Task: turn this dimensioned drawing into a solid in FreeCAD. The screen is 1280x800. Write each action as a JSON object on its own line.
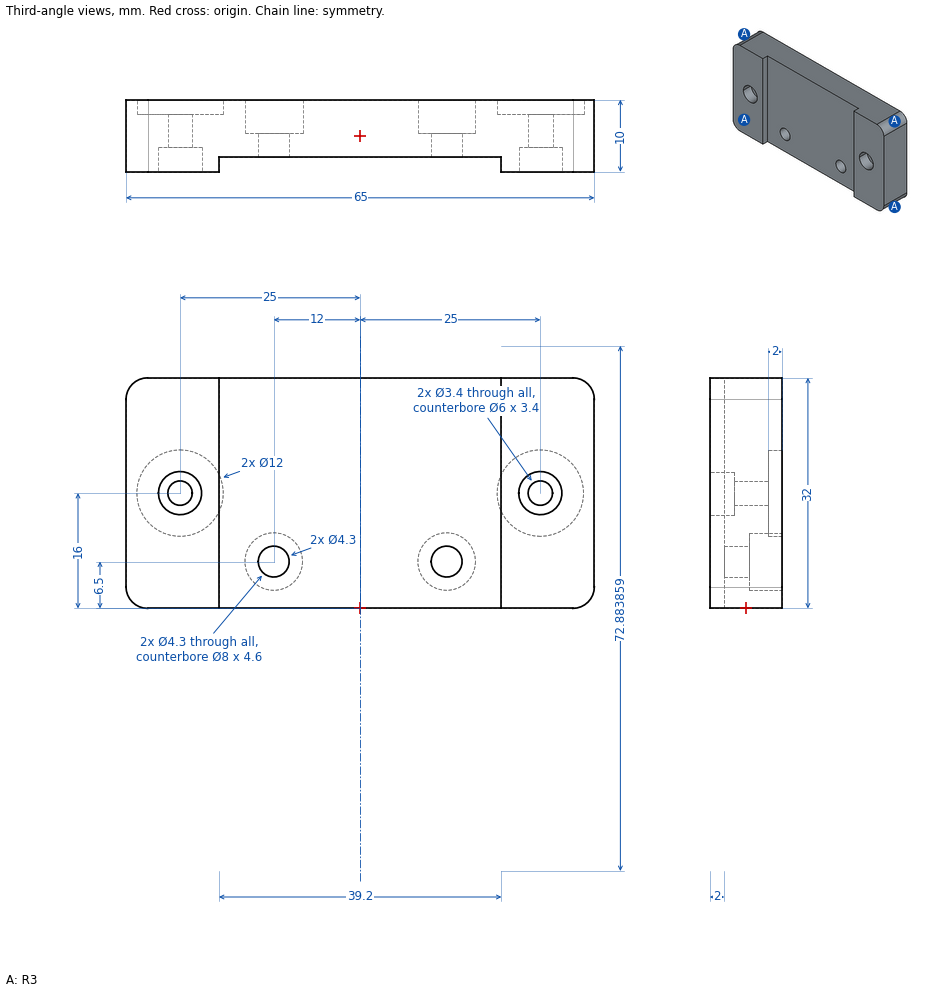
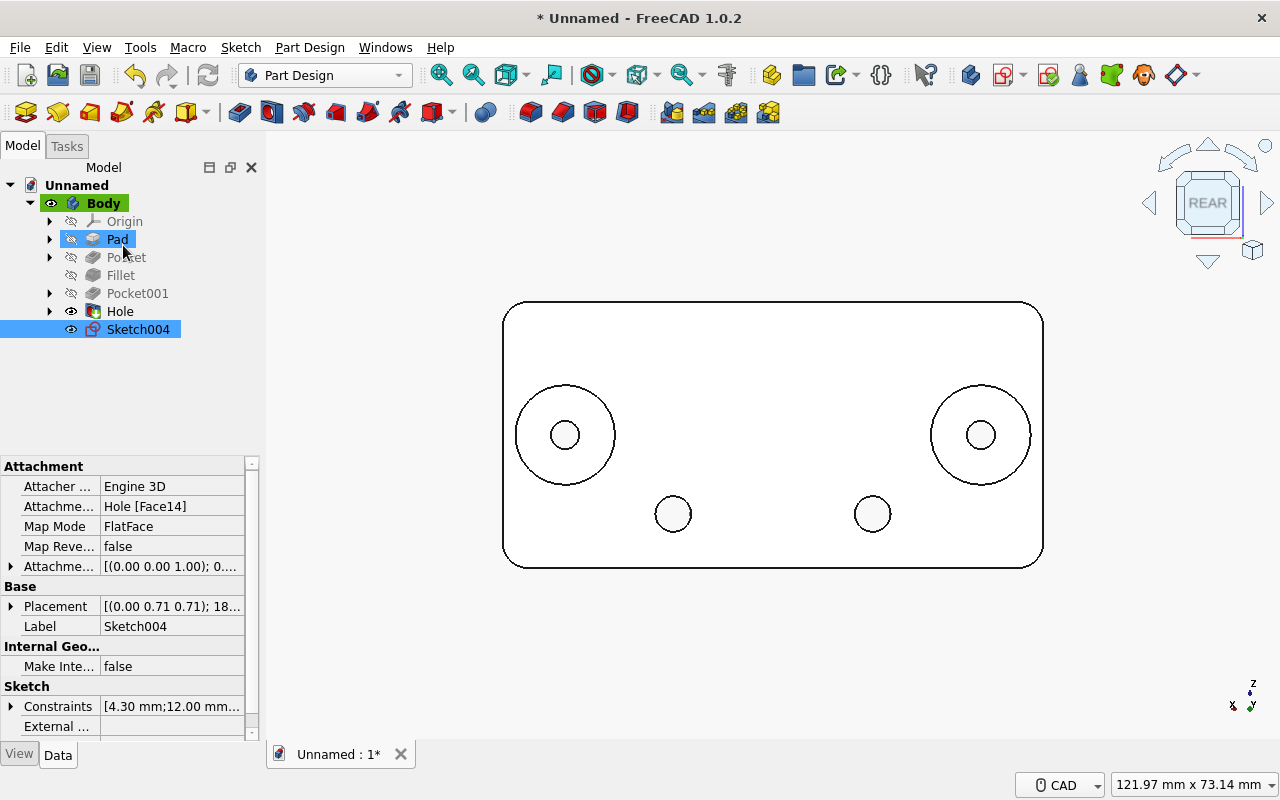
{"action": "left_click", "coordinate": [272, 112]}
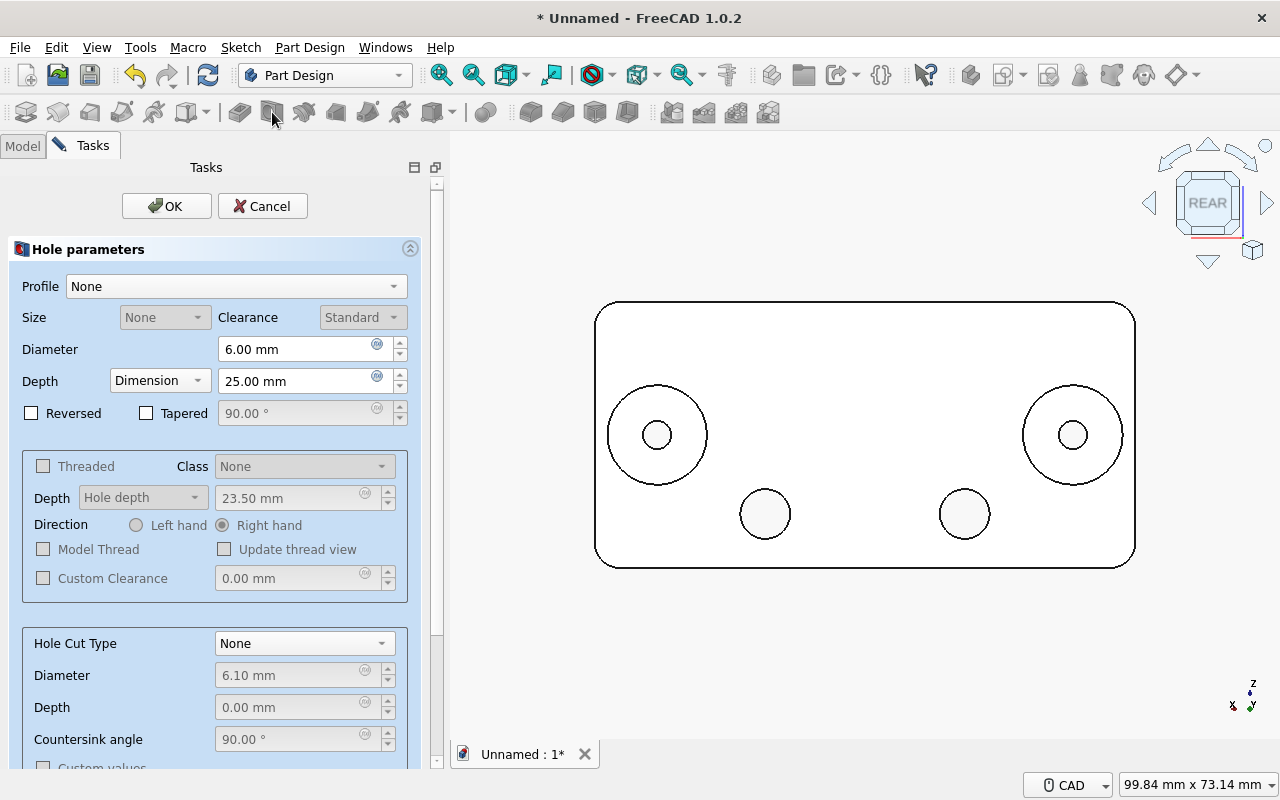
{"action": "triple_click", "coordinate": [305, 349]}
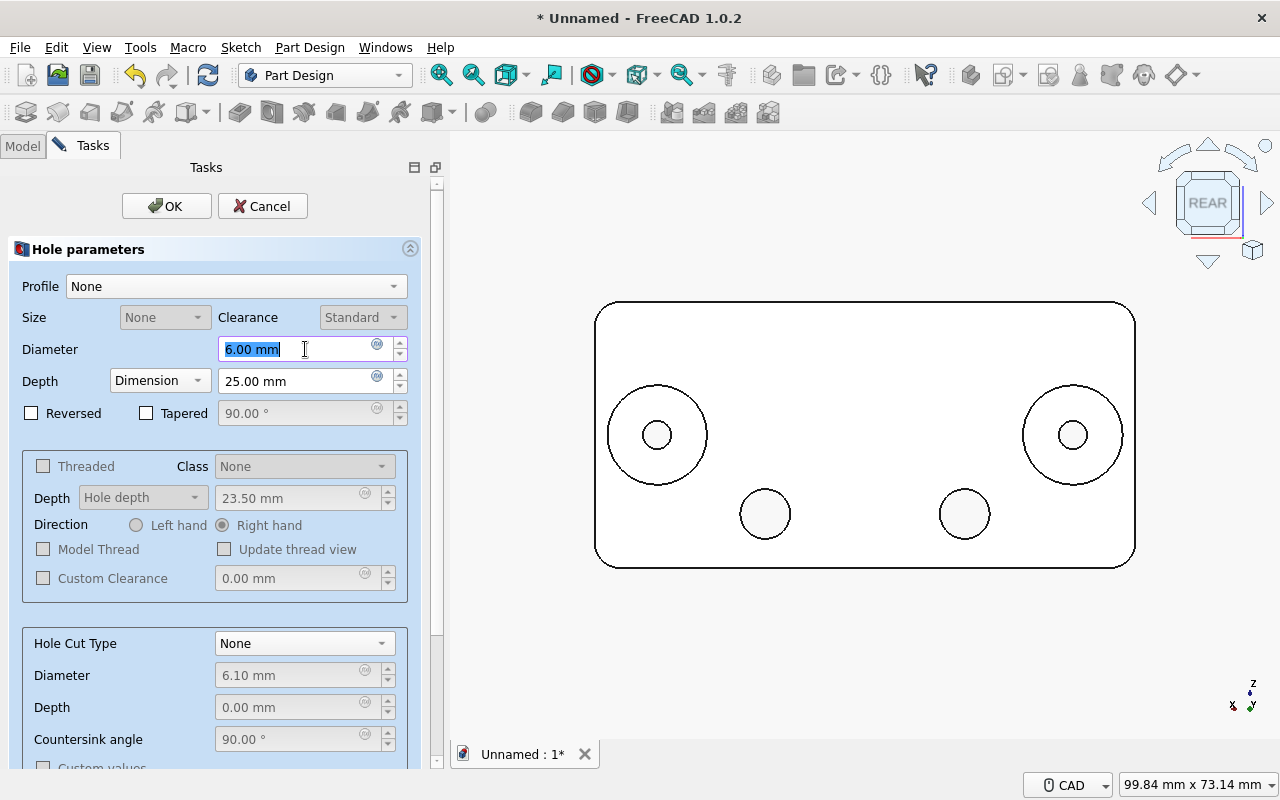
{"action": "type", "text": "4.3"}
{"action": "key", "text": "Tab"}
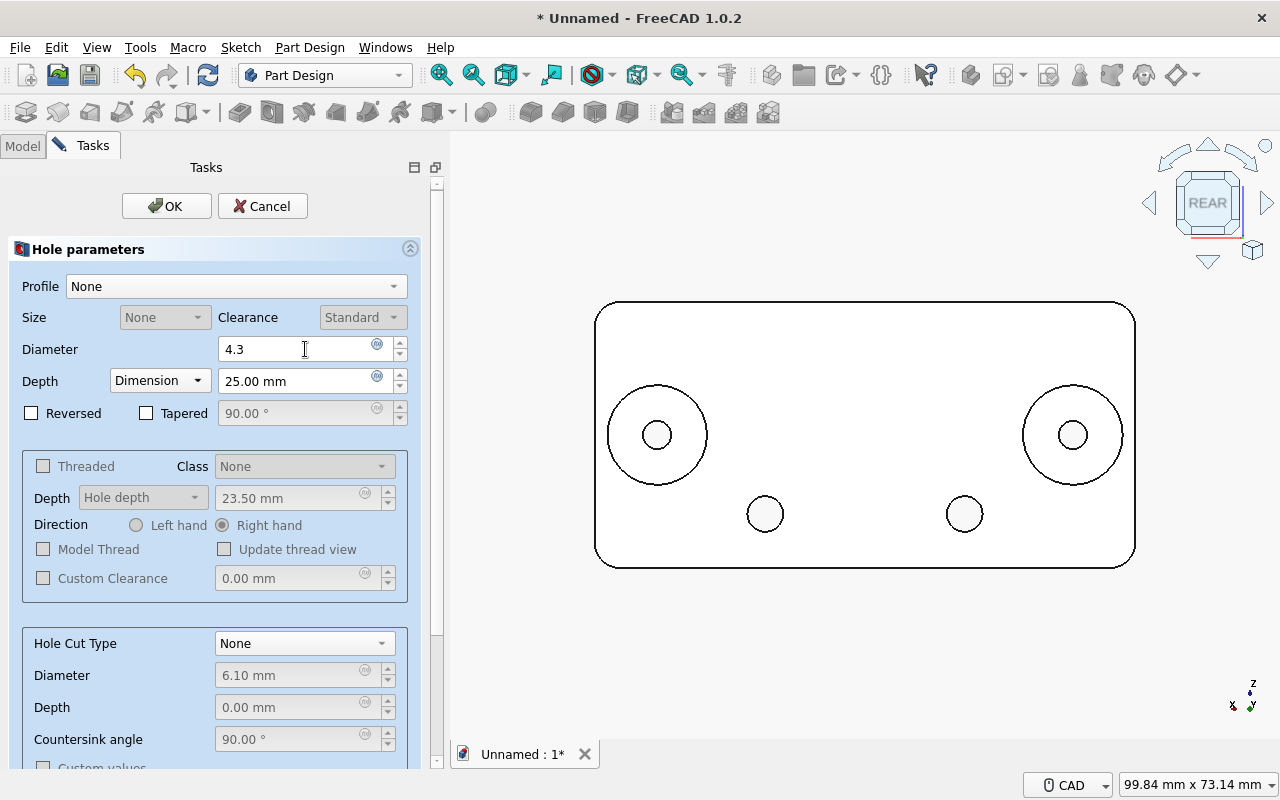
{"action": "left_click", "coordinate": [161, 380]}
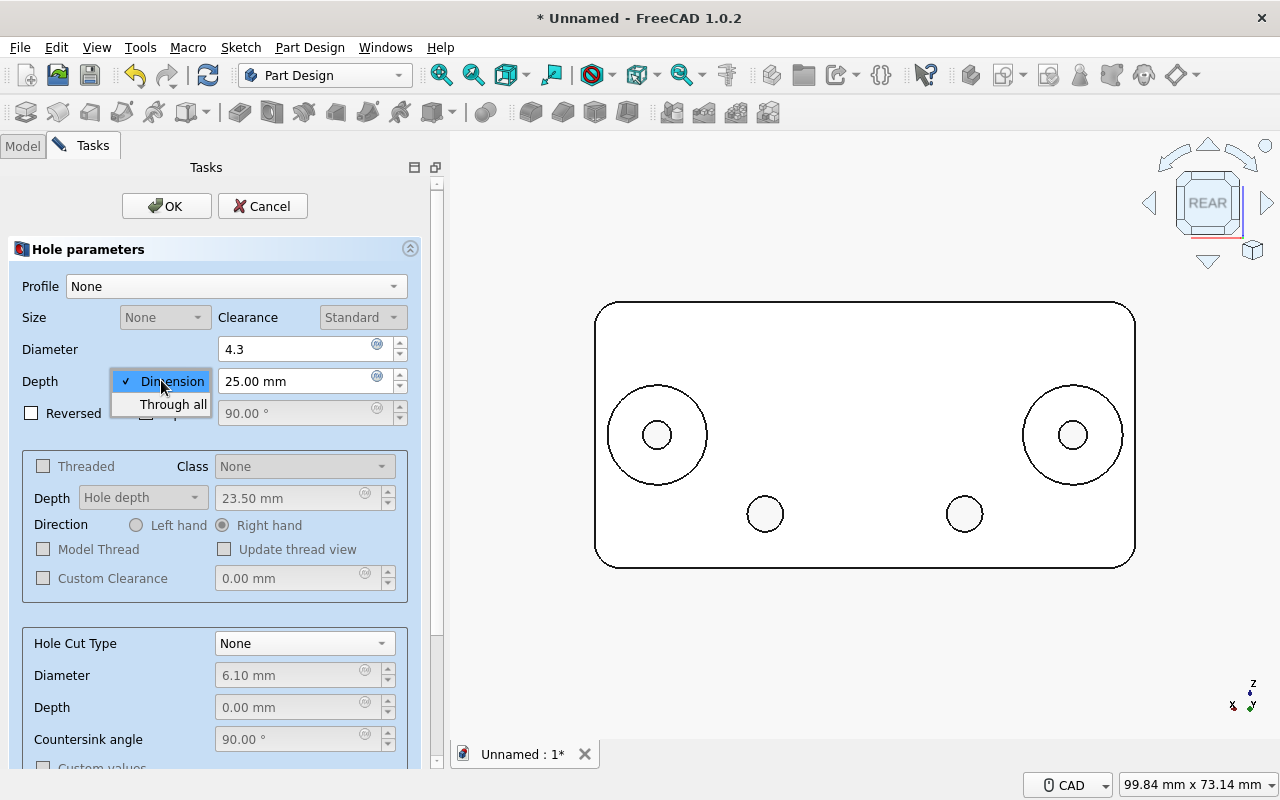
{"action": "left_click", "coordinate": [160, 404]}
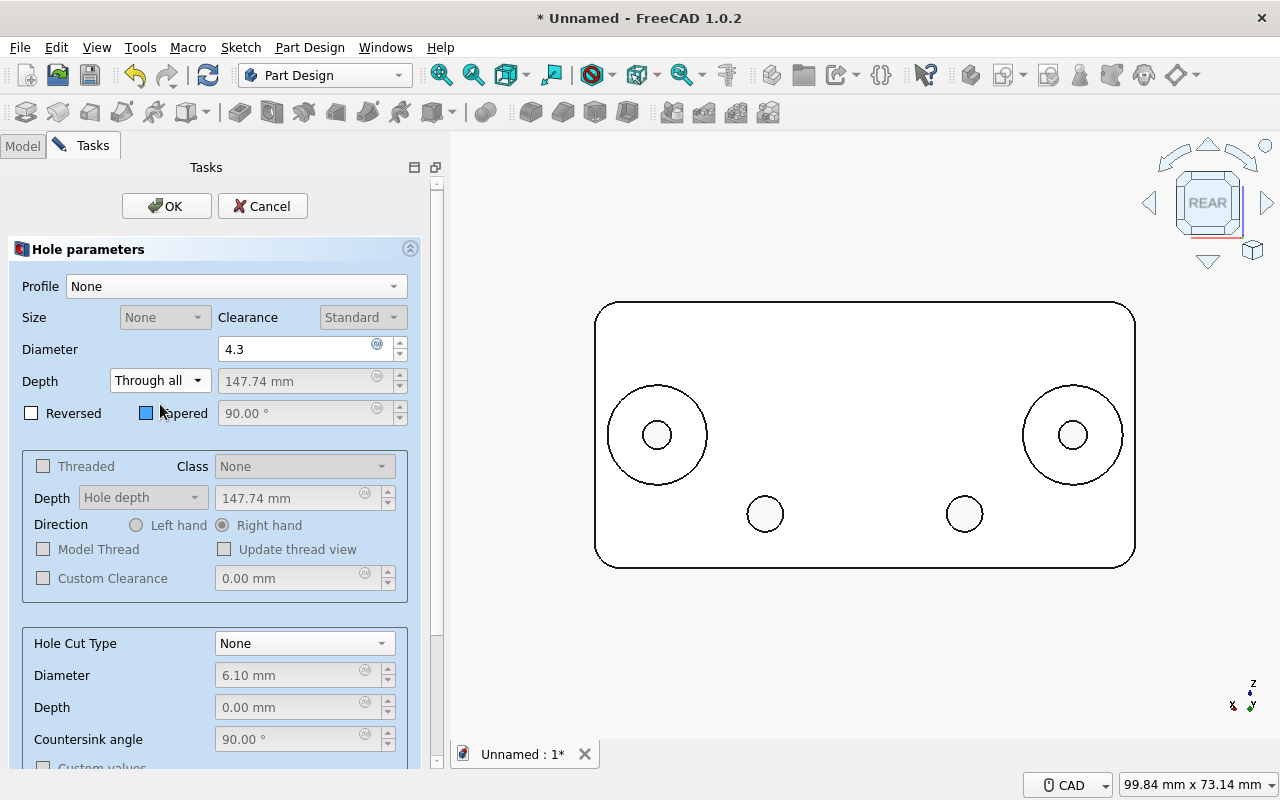
{"action": "left_click", "coordinate": [306, 644]}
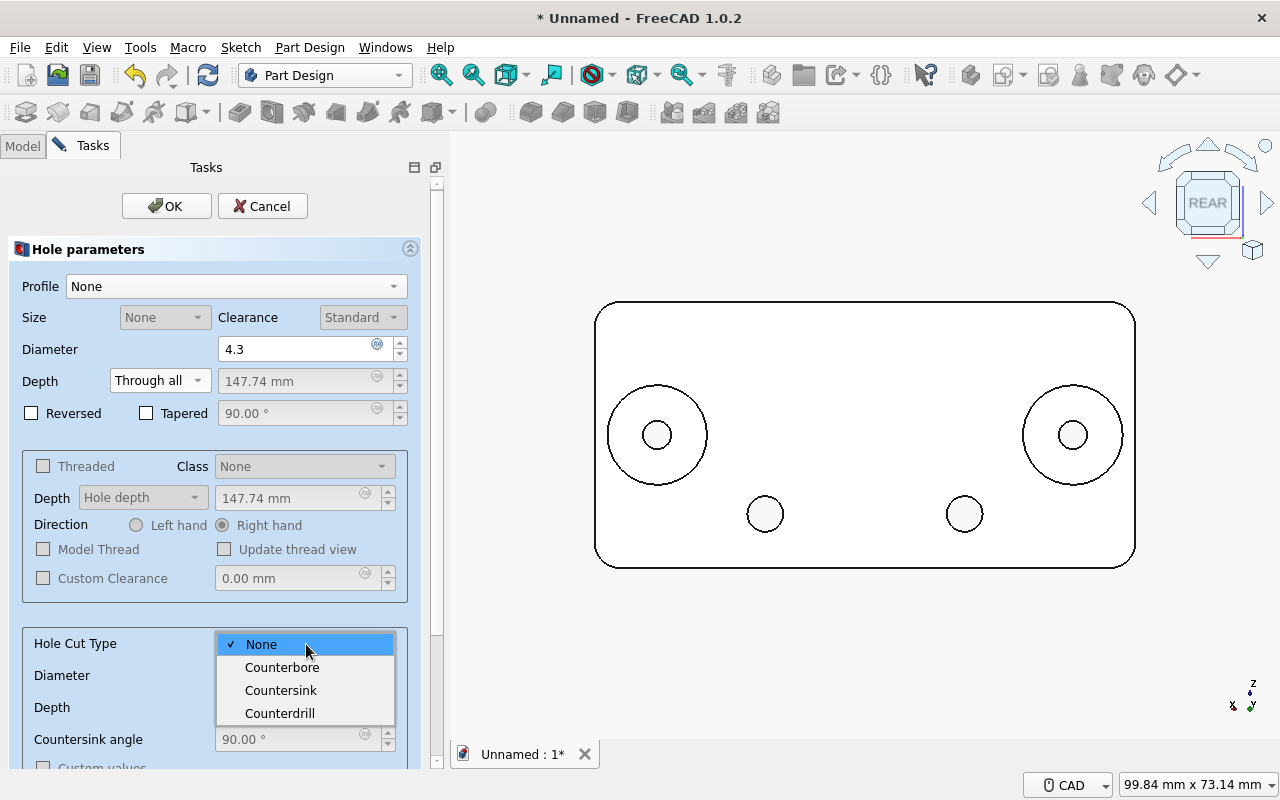
{"action": "left_click", "coordinate": [304, 668]}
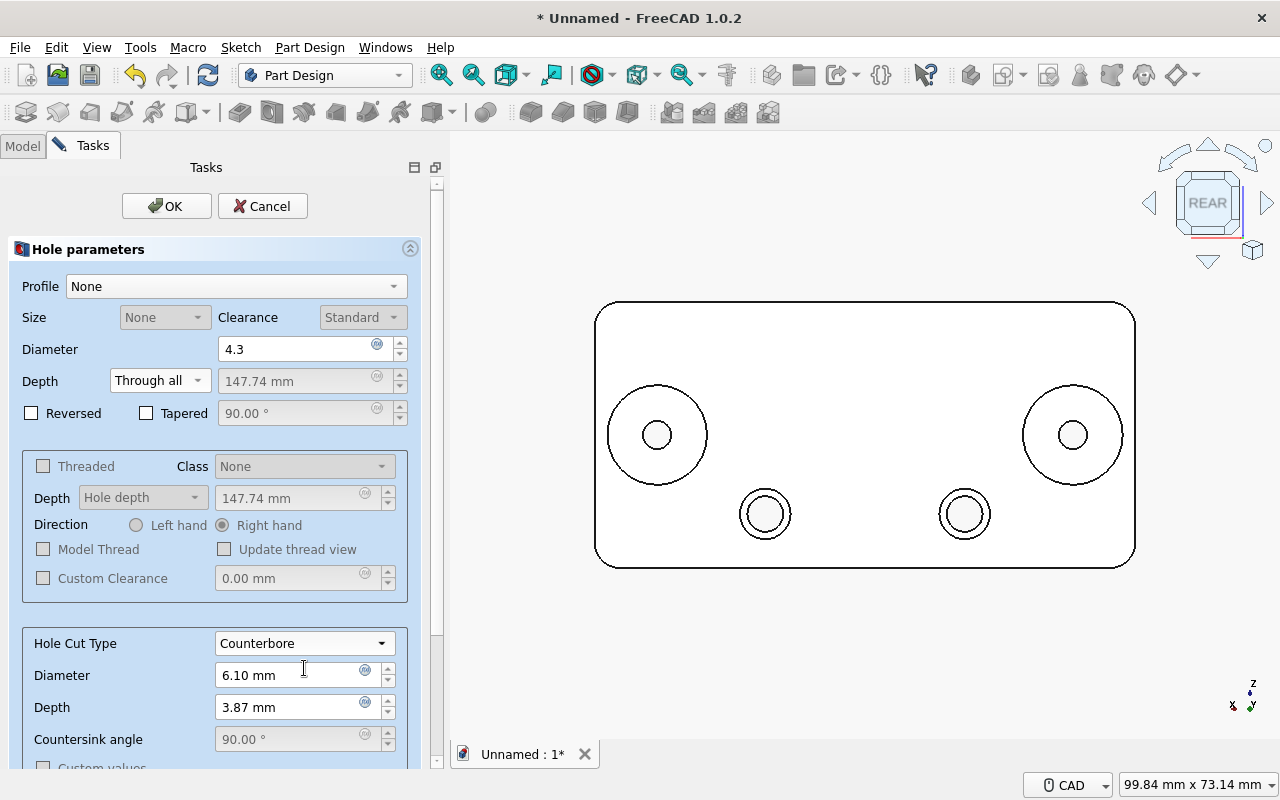
{"action": "triple_click", "coordinate": [298, 675]}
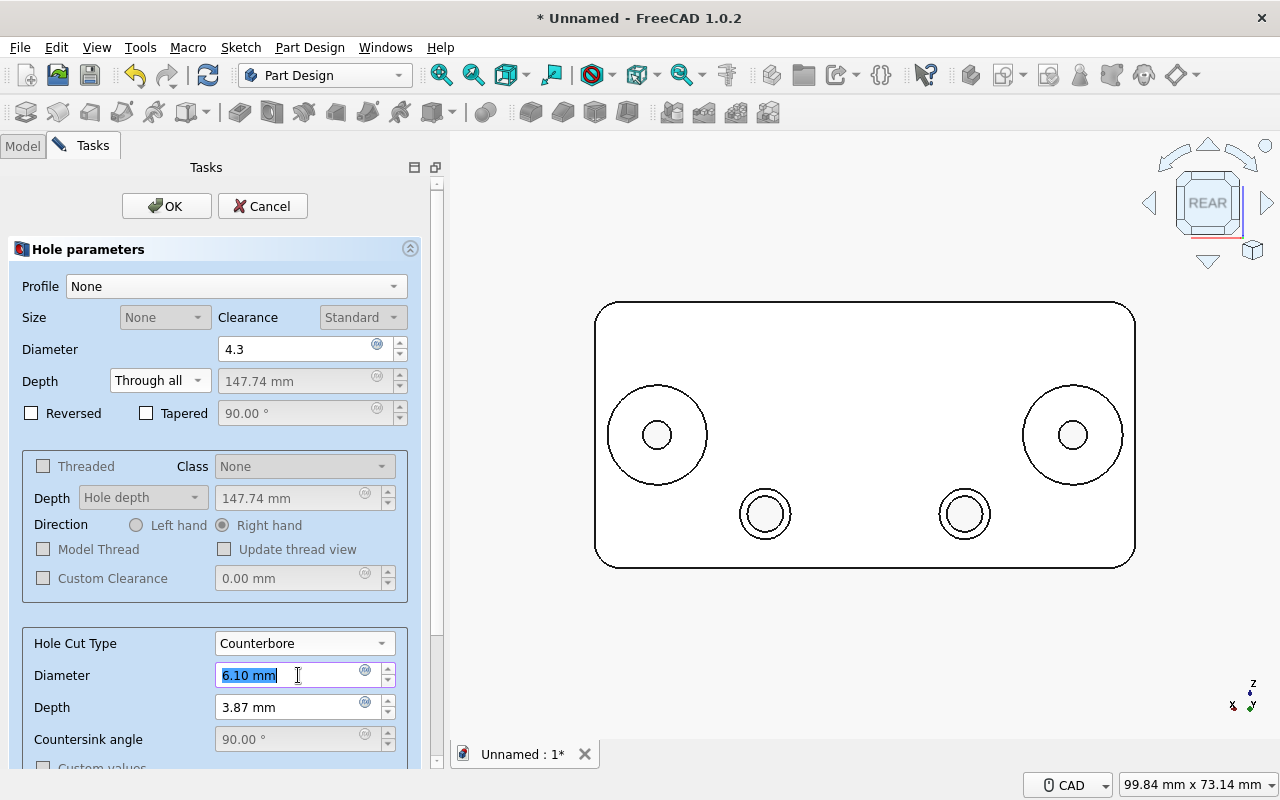
{"action": "type", "text": "8"}
{"action": "key", "text": "Tab"}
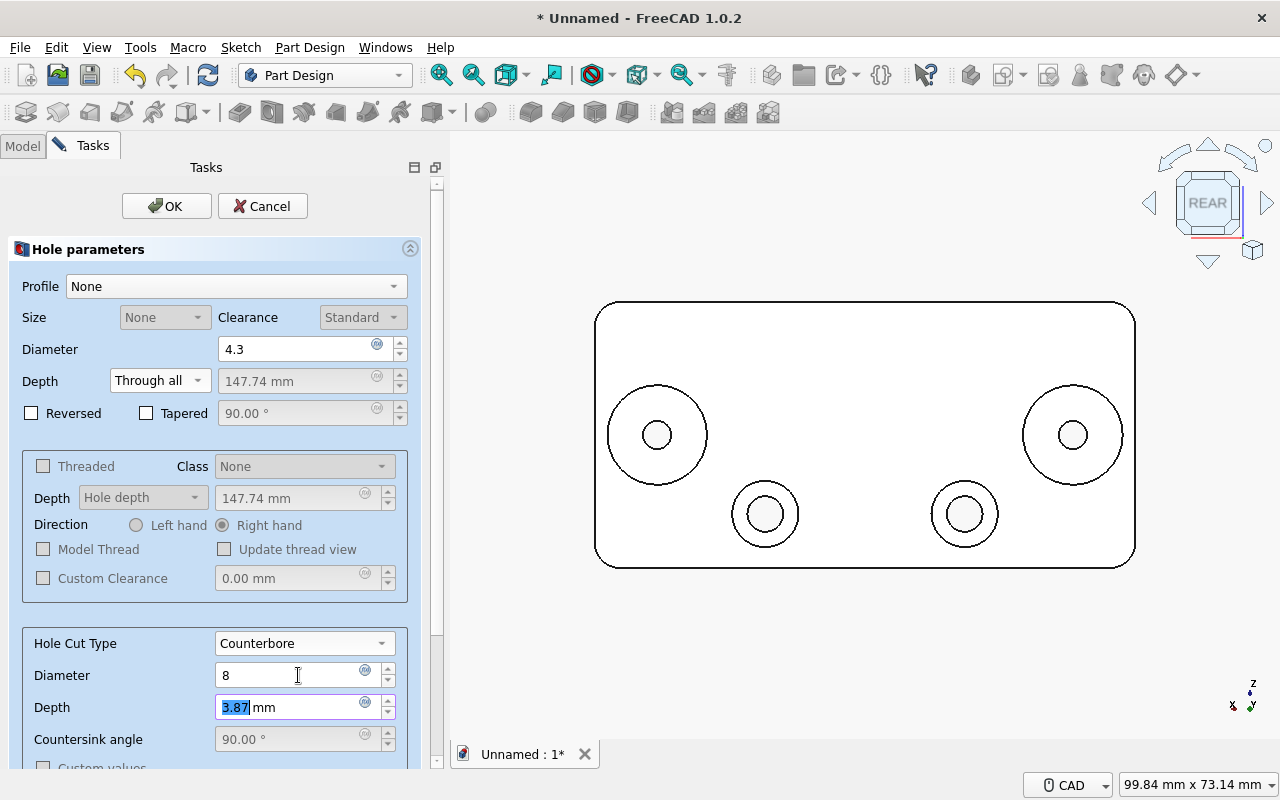
{"action": "type", "text": "4.6"}
{"action": "key", "text": "Tab"}